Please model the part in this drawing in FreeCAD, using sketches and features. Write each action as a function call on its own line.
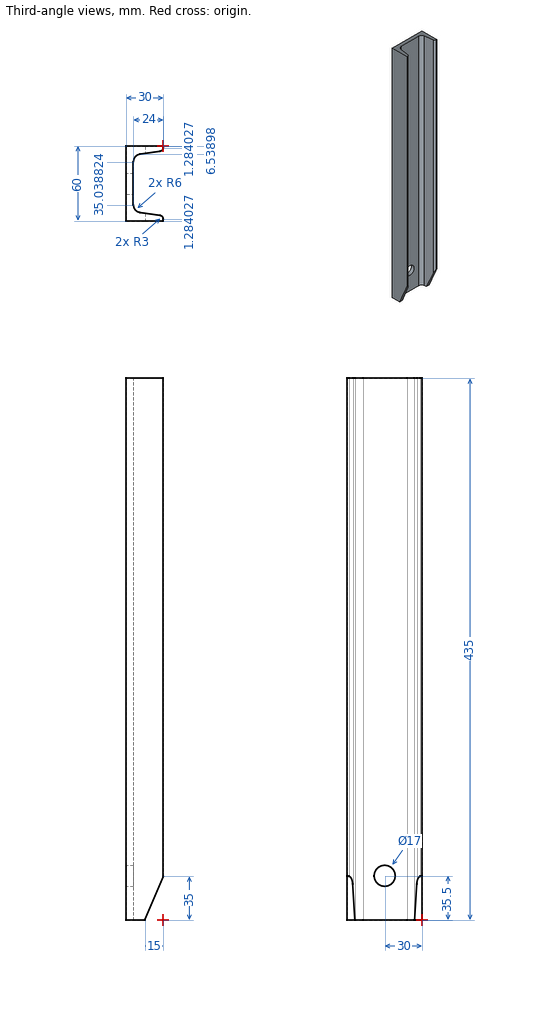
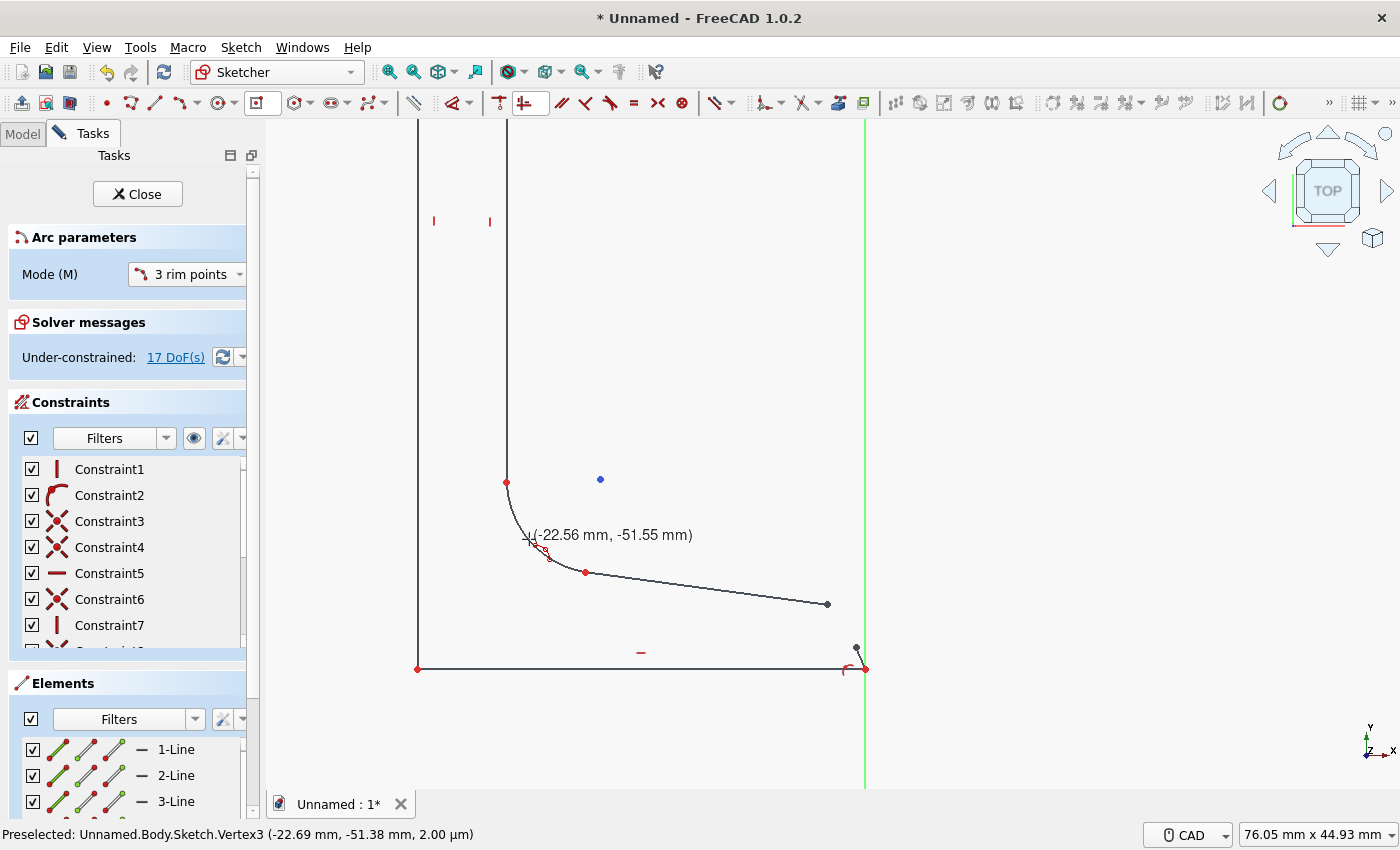
scroll(865, 646, down, 4)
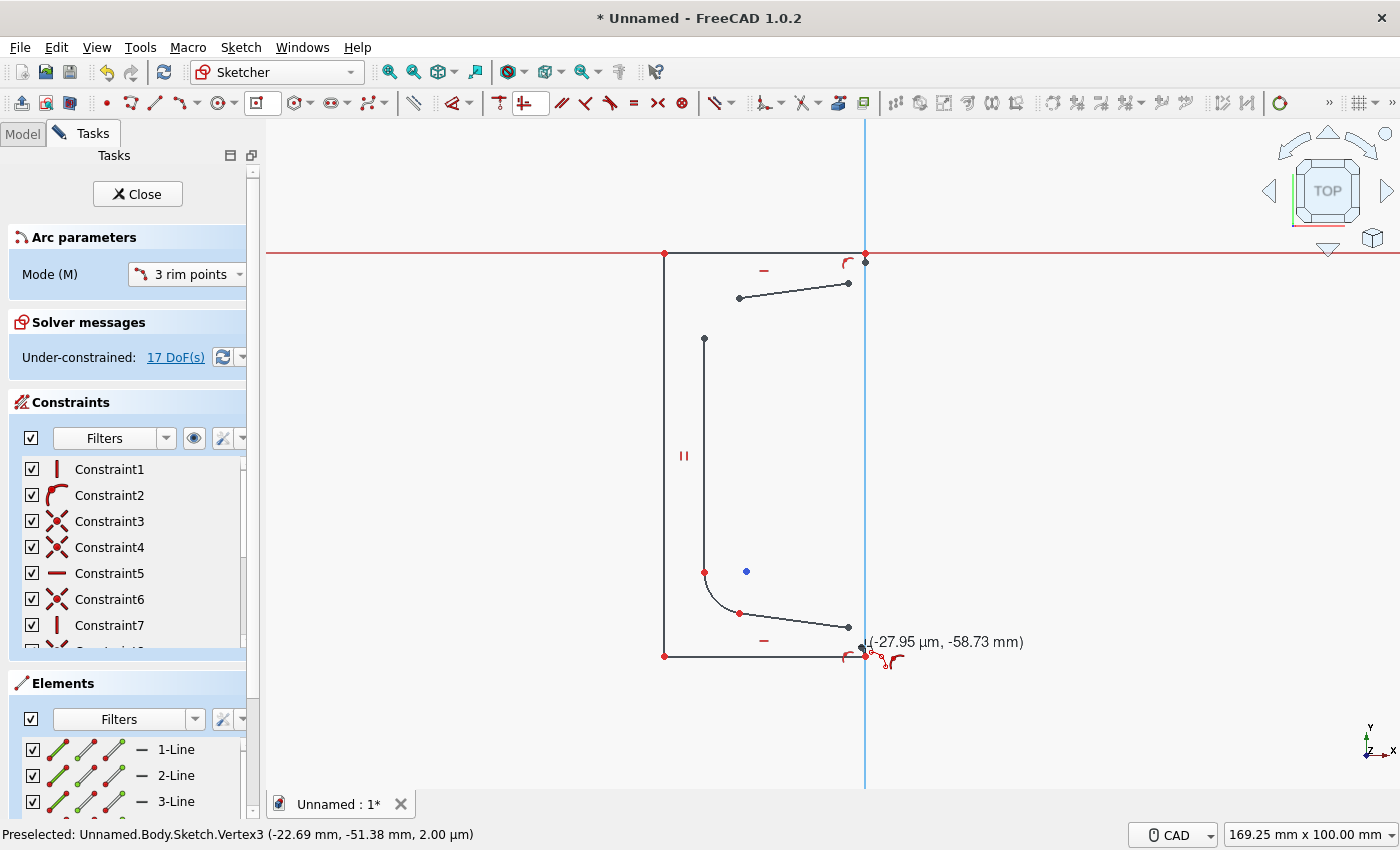
click(704, 338)
click(740, 298)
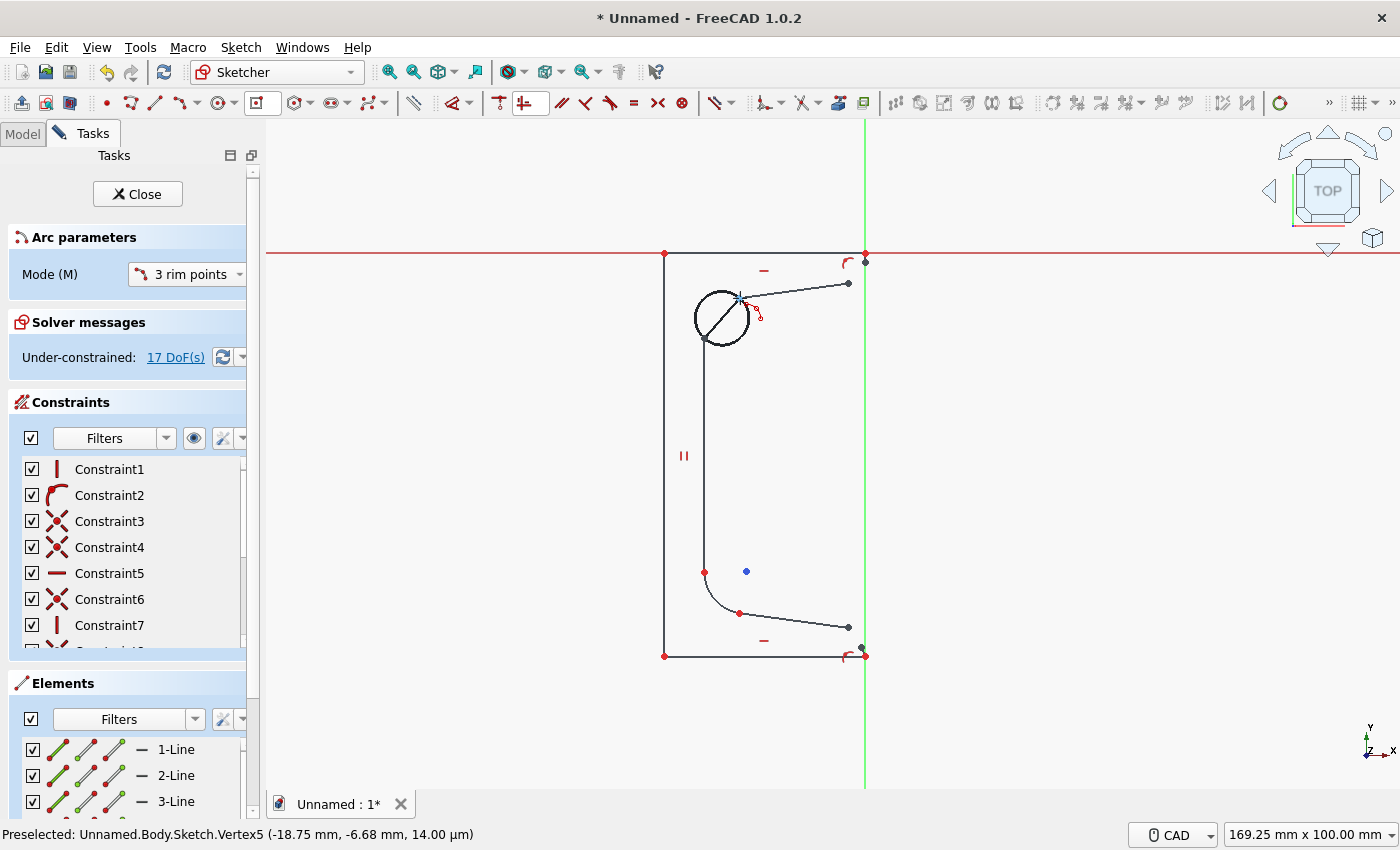
scroll(715, 311, up, 3)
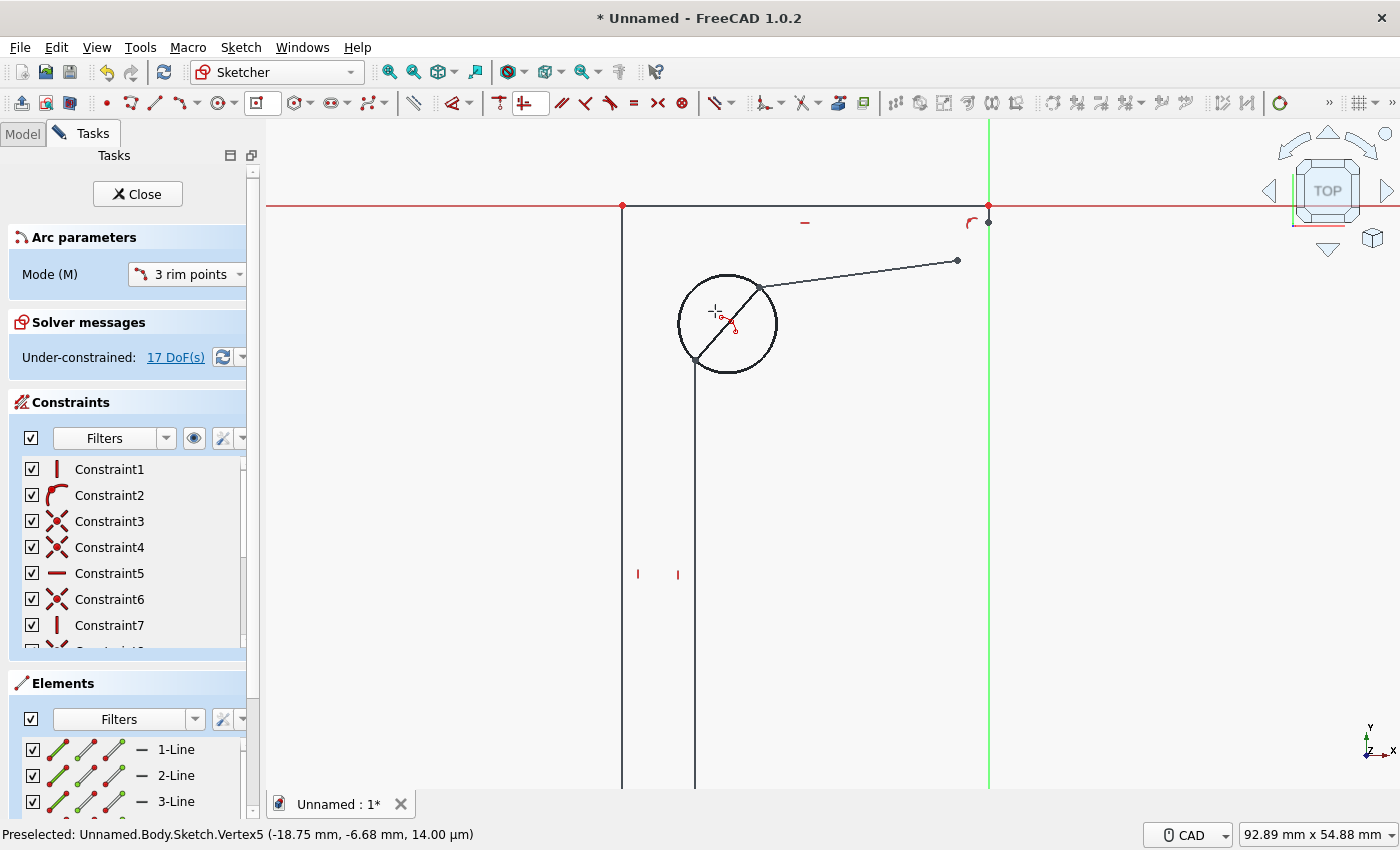
click(714, 310)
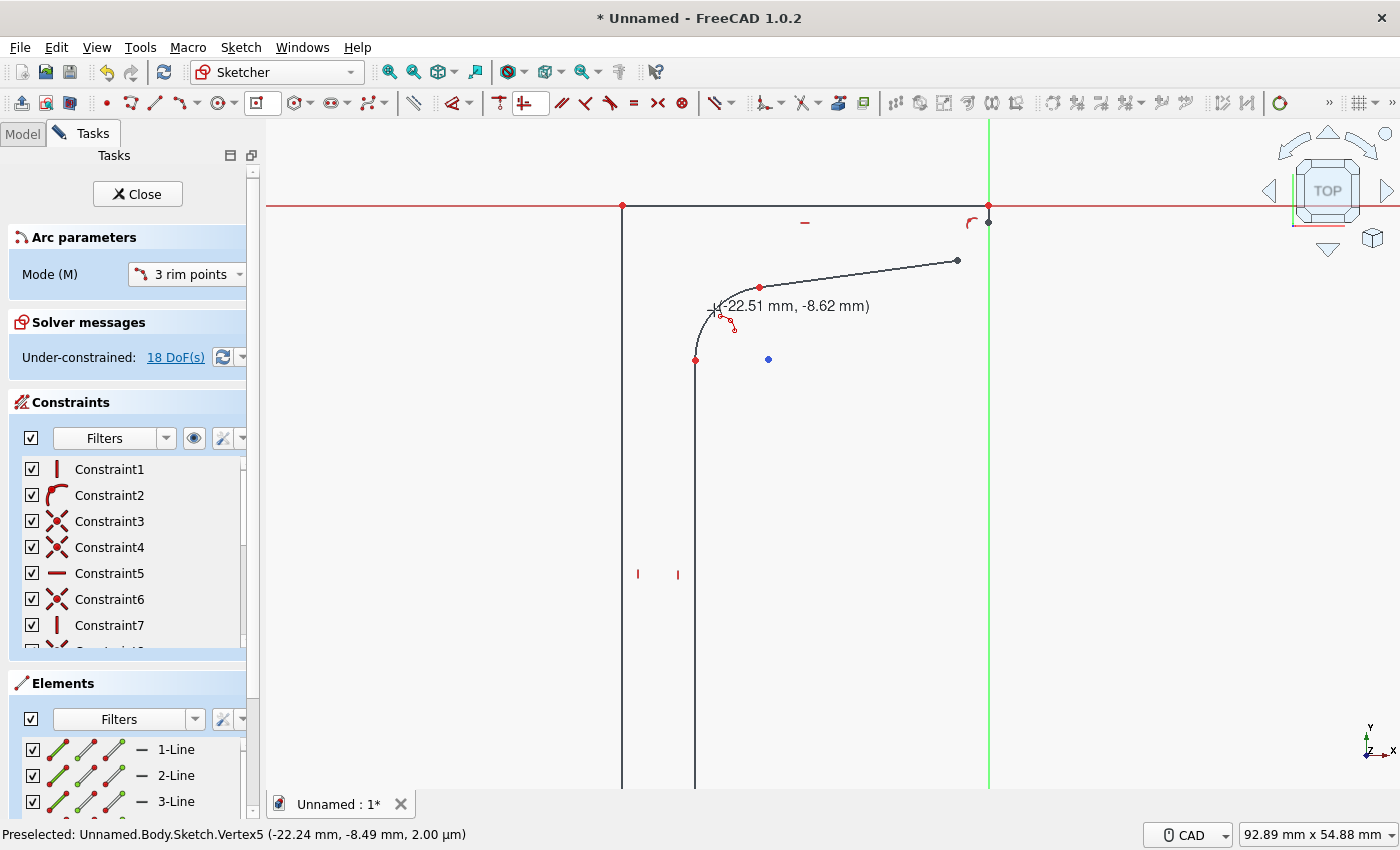
click(958, 261)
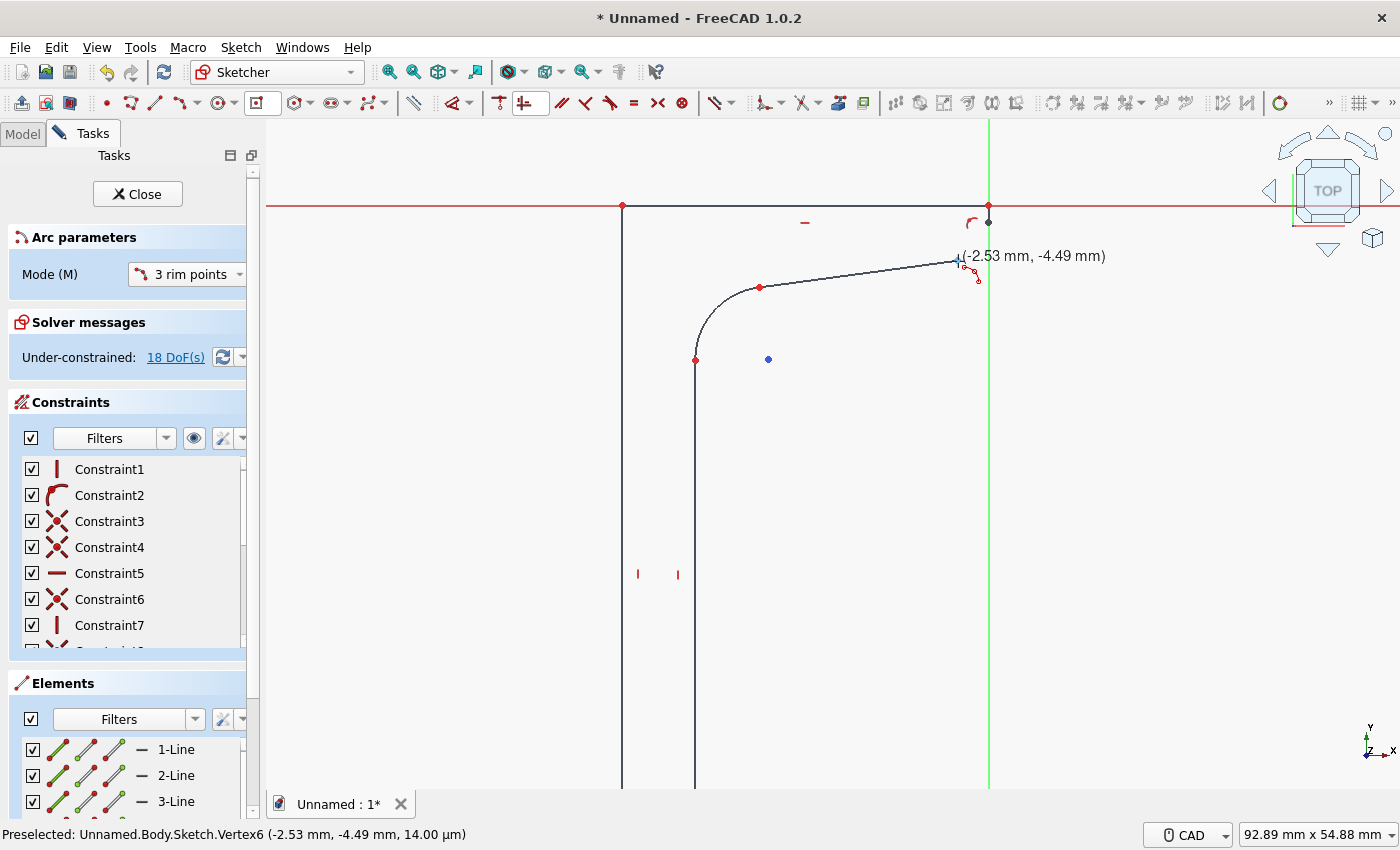
scroll(989, 221, up, 4)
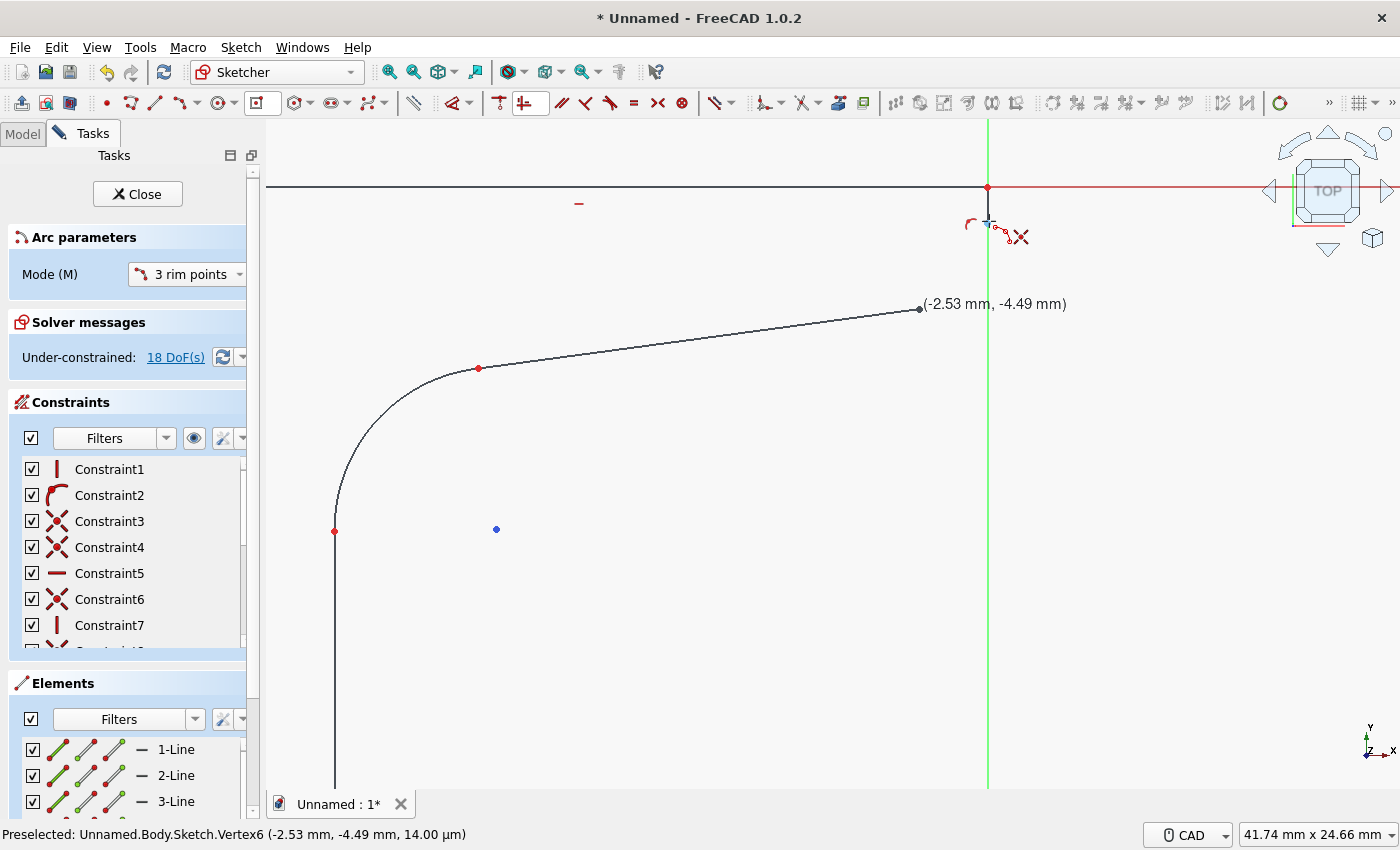
click(988, 223)
click(968, 275)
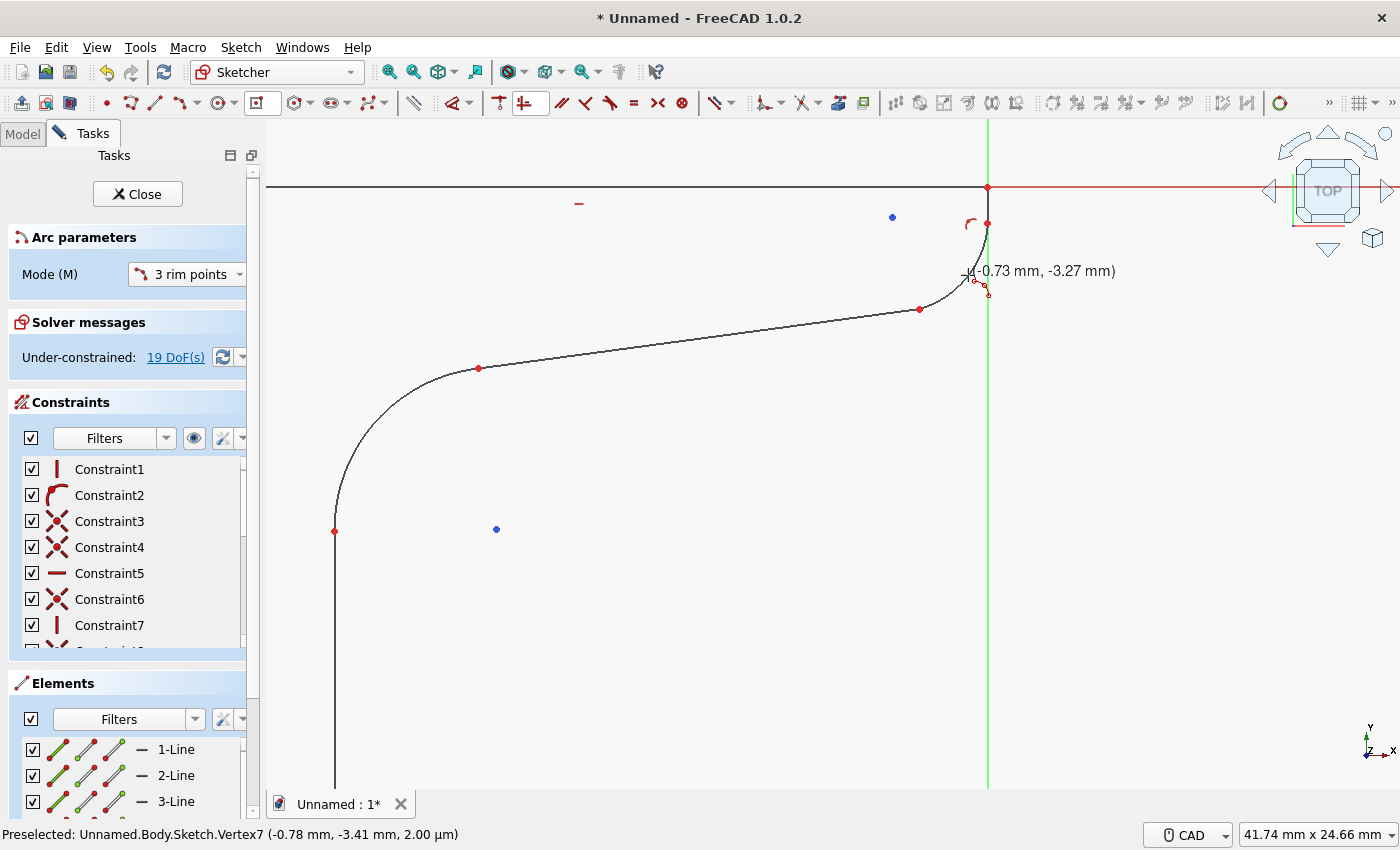
scroll(825, 275, down, 7)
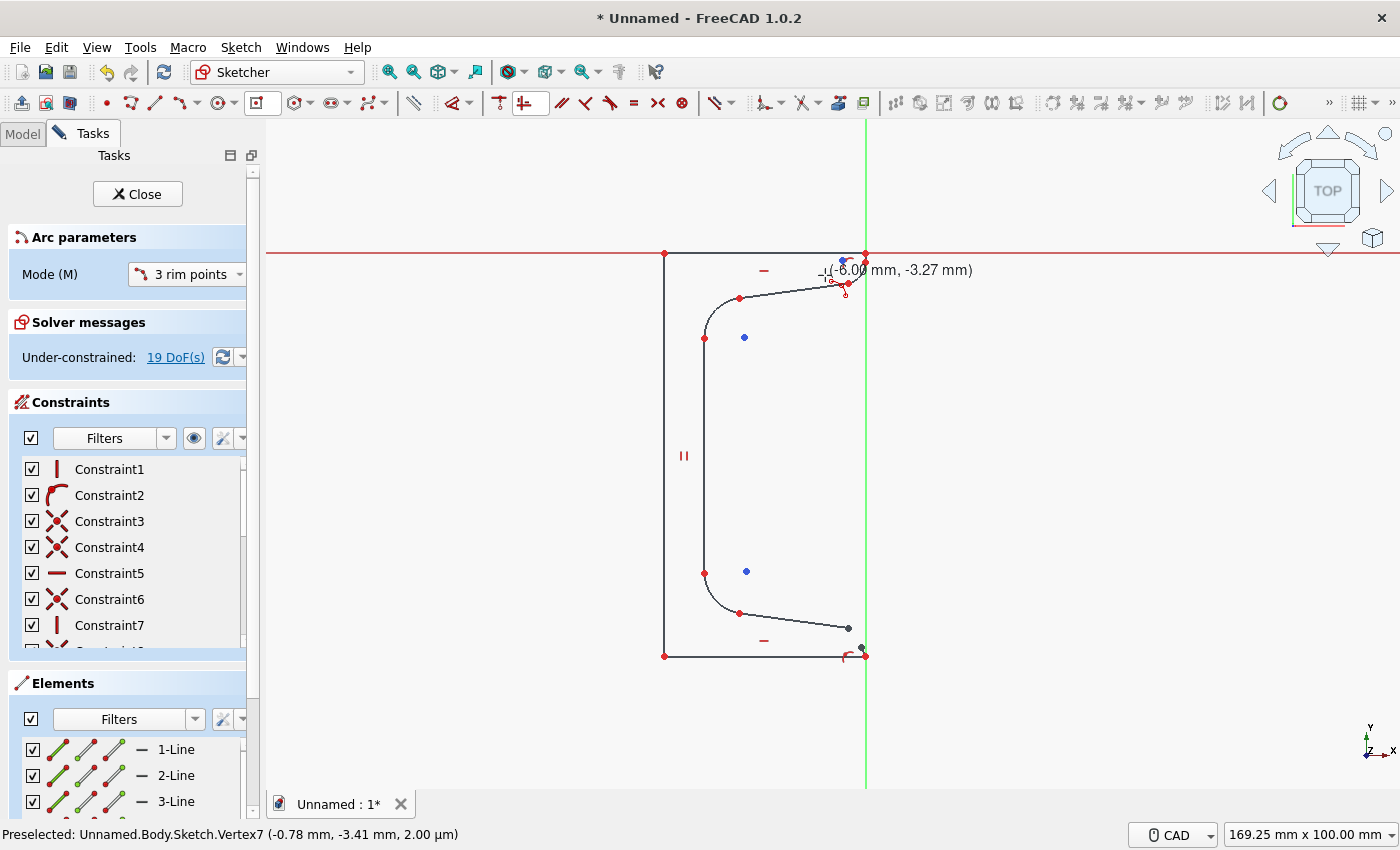
scroll(866, 647, up, 7)